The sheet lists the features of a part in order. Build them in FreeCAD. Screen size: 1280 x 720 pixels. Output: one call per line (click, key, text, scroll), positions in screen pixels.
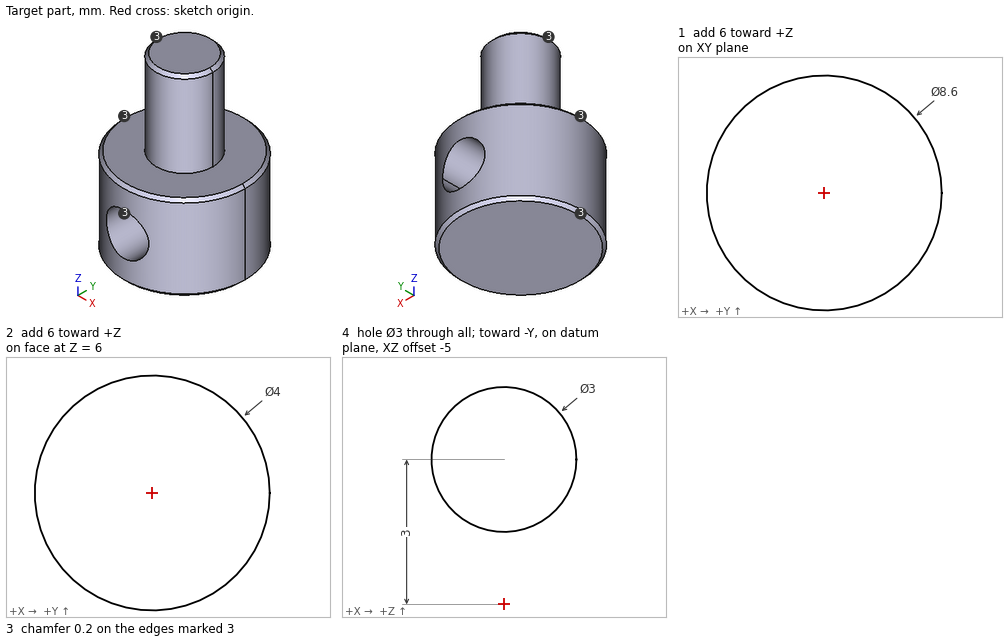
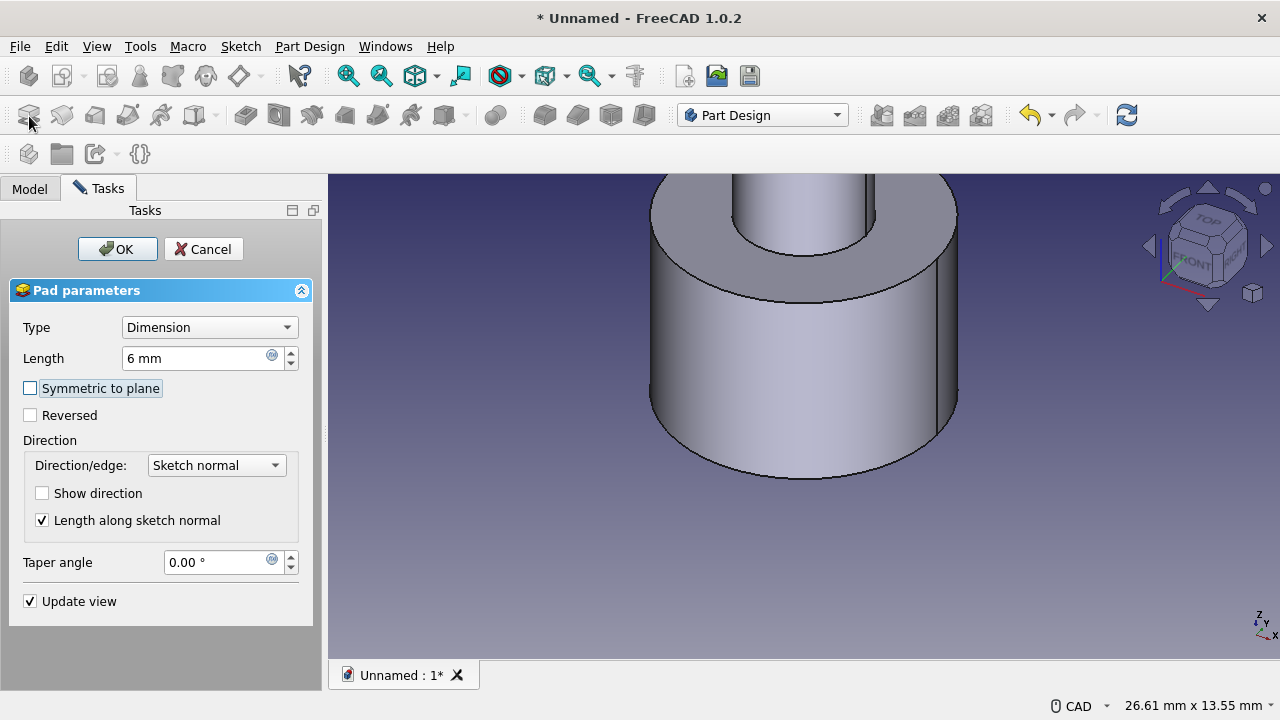
click(118, 249)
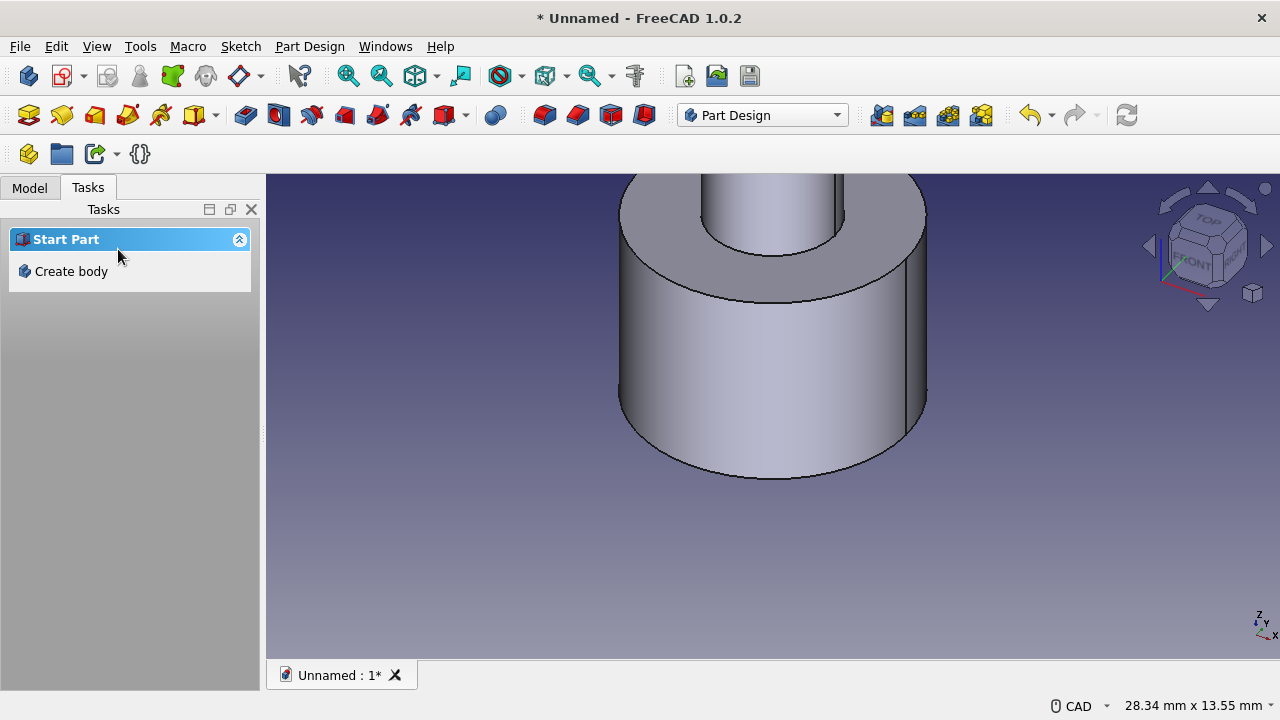
key(v)
key(f)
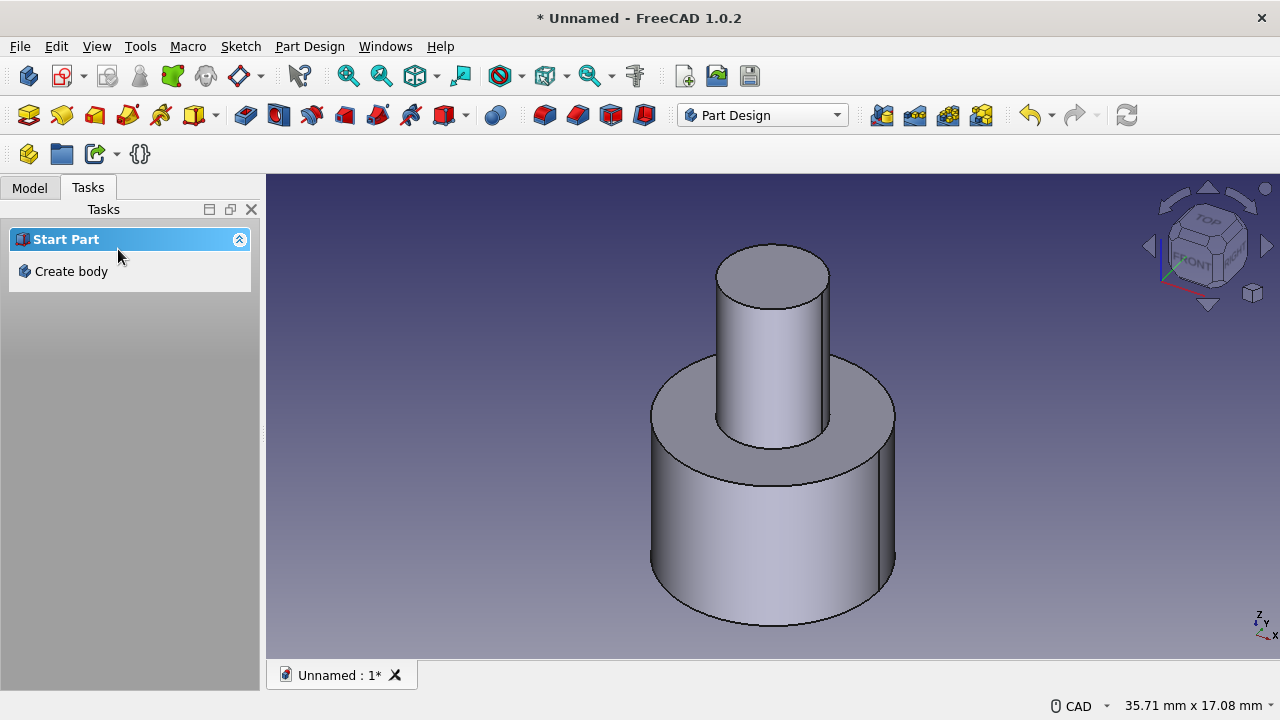
click(651, 423)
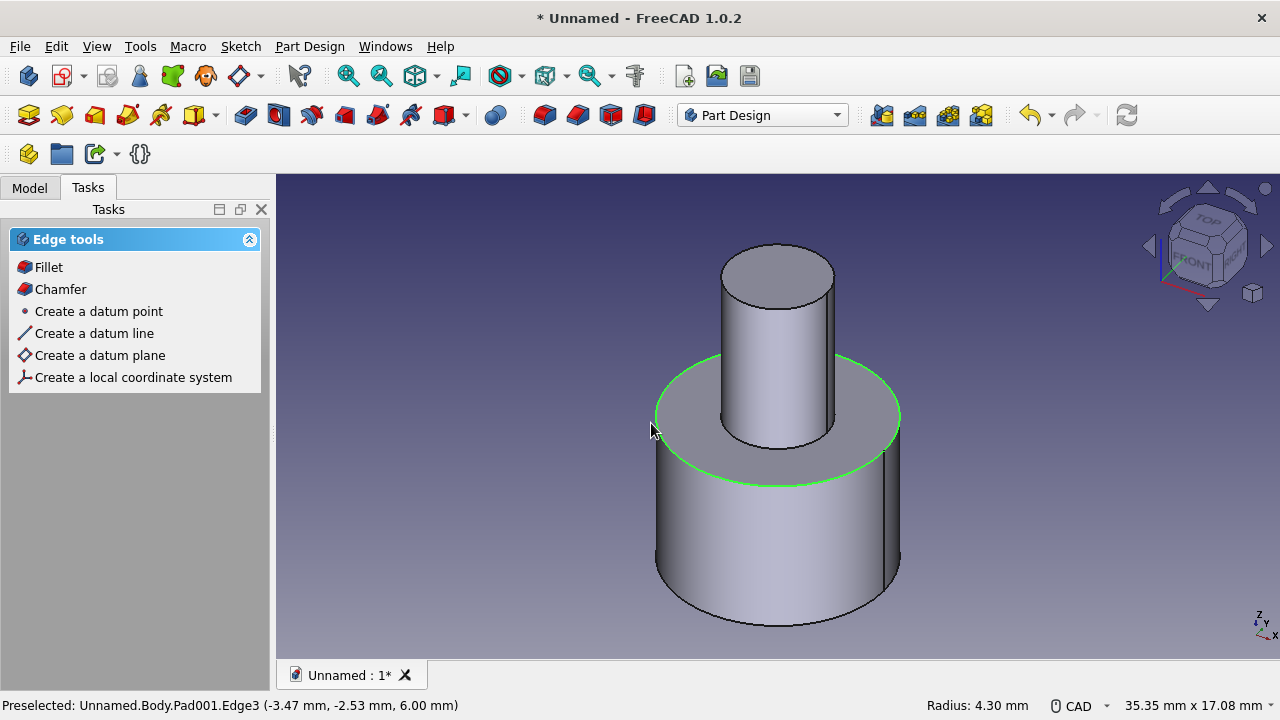
click(721, 279, ctrl)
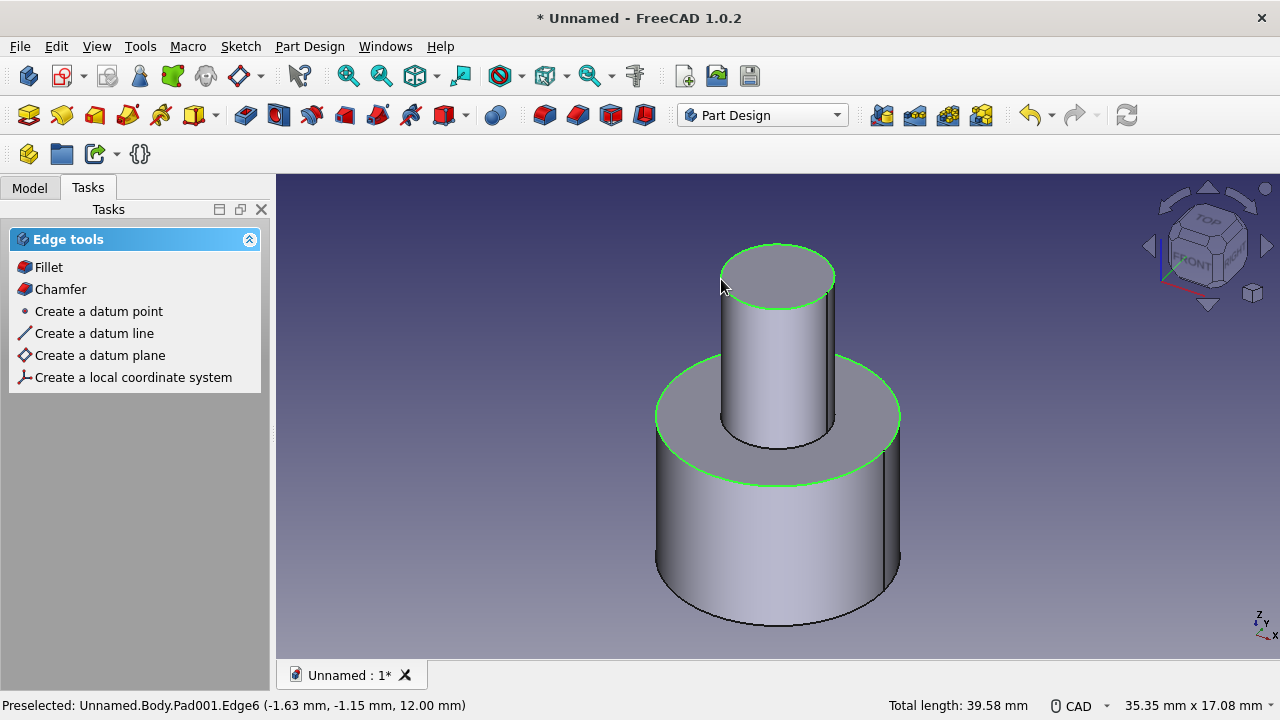
key(0)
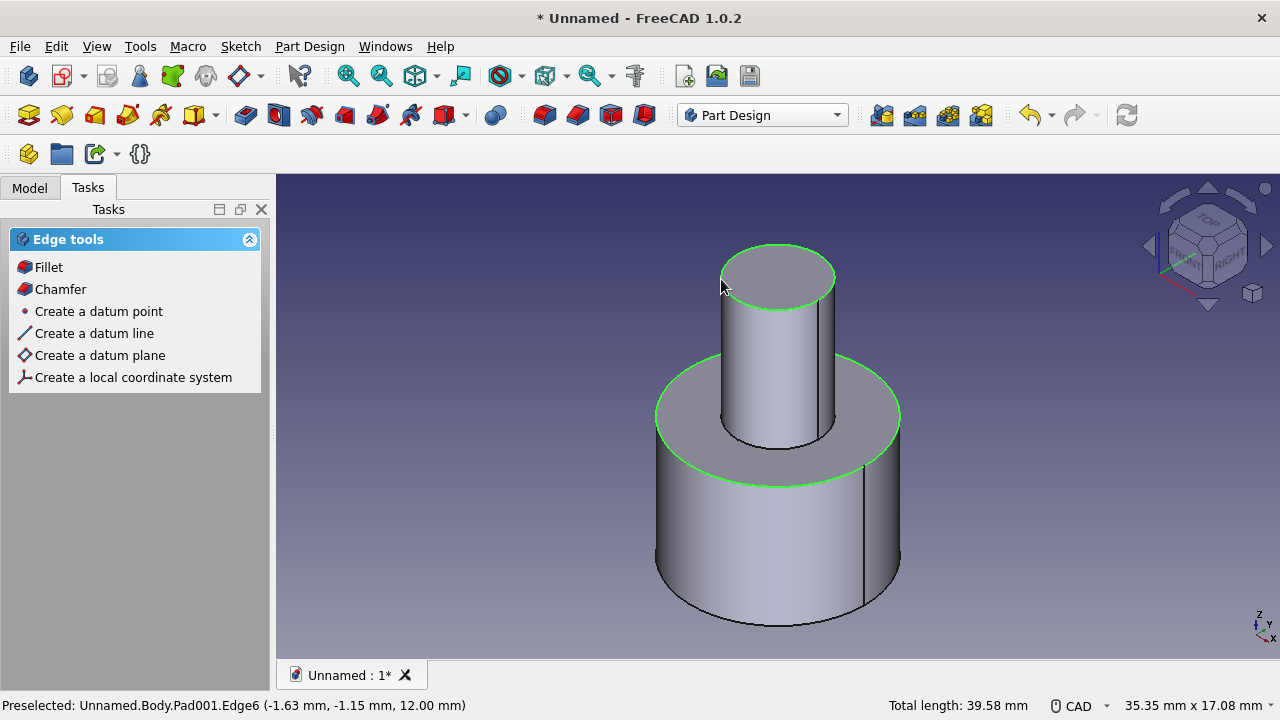
key(2)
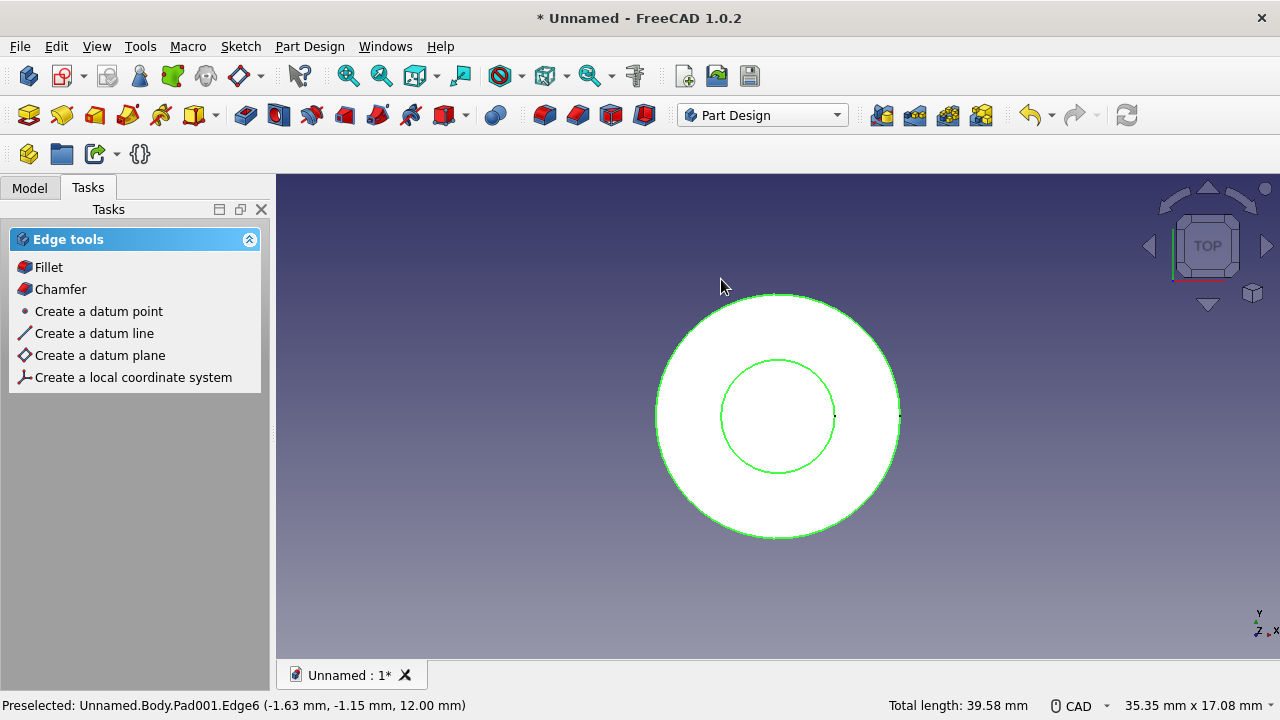
key(1)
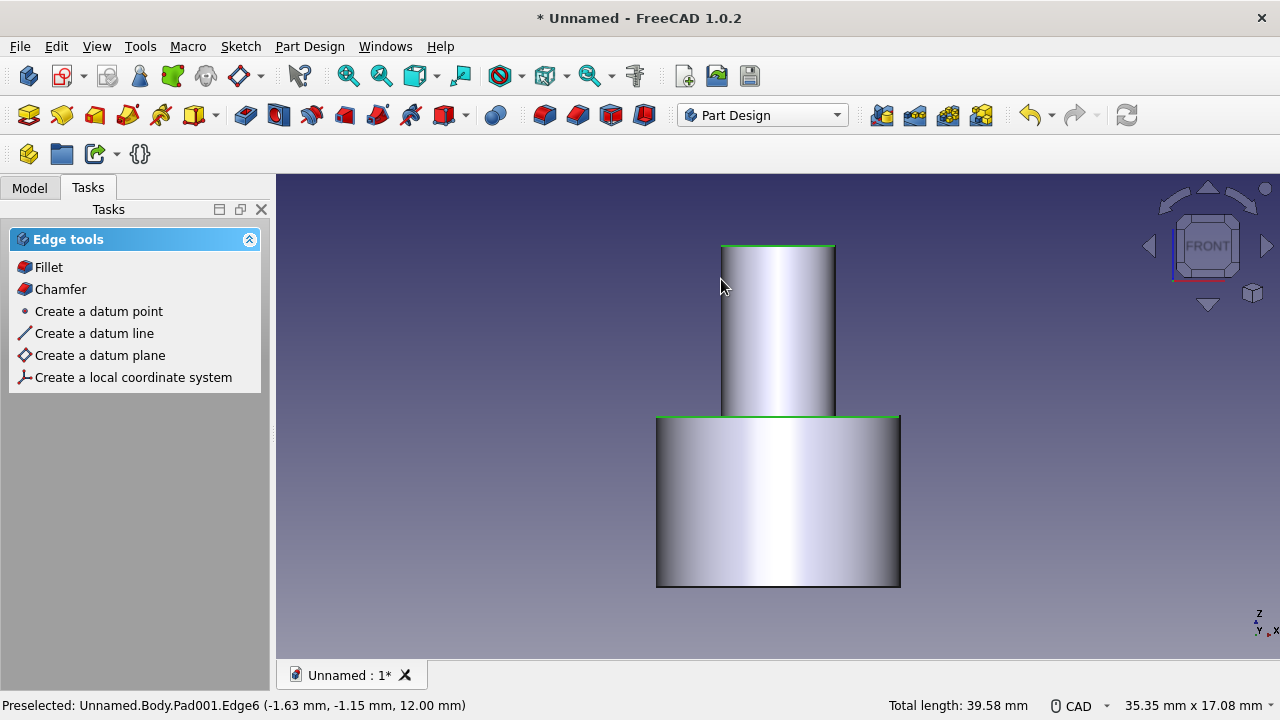
click(679, 586, ctrl)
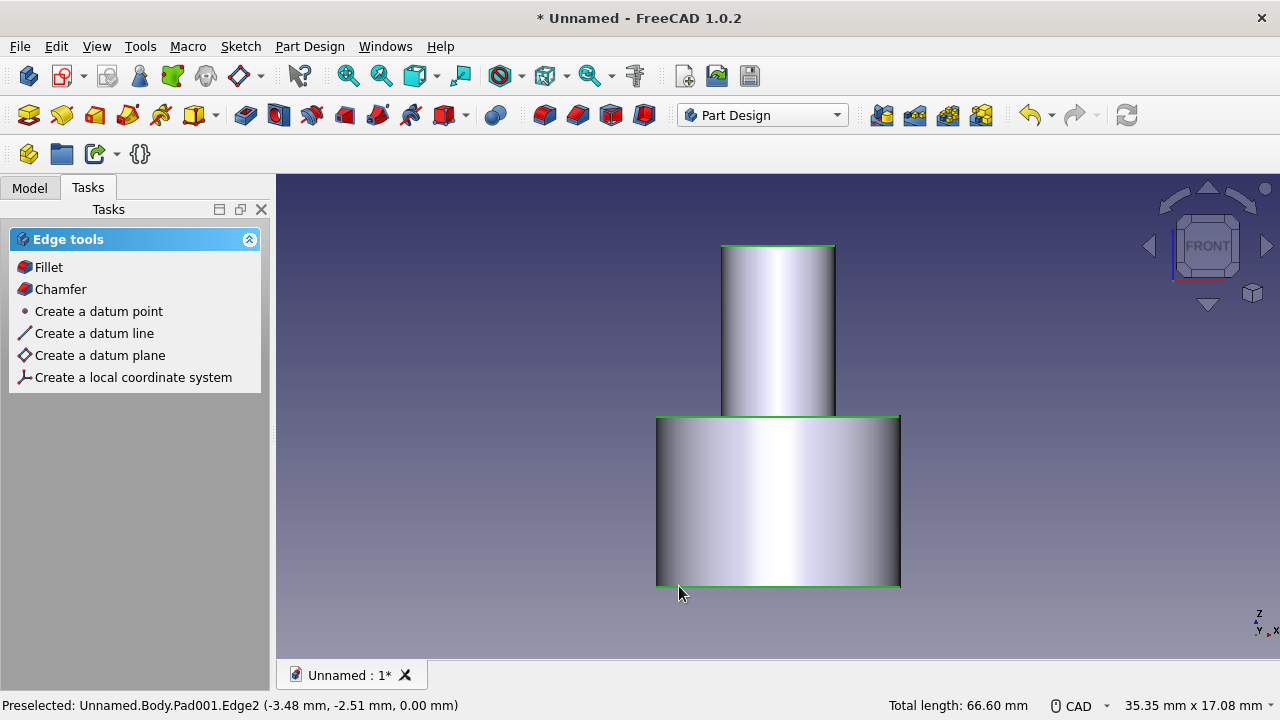
click(578, 116)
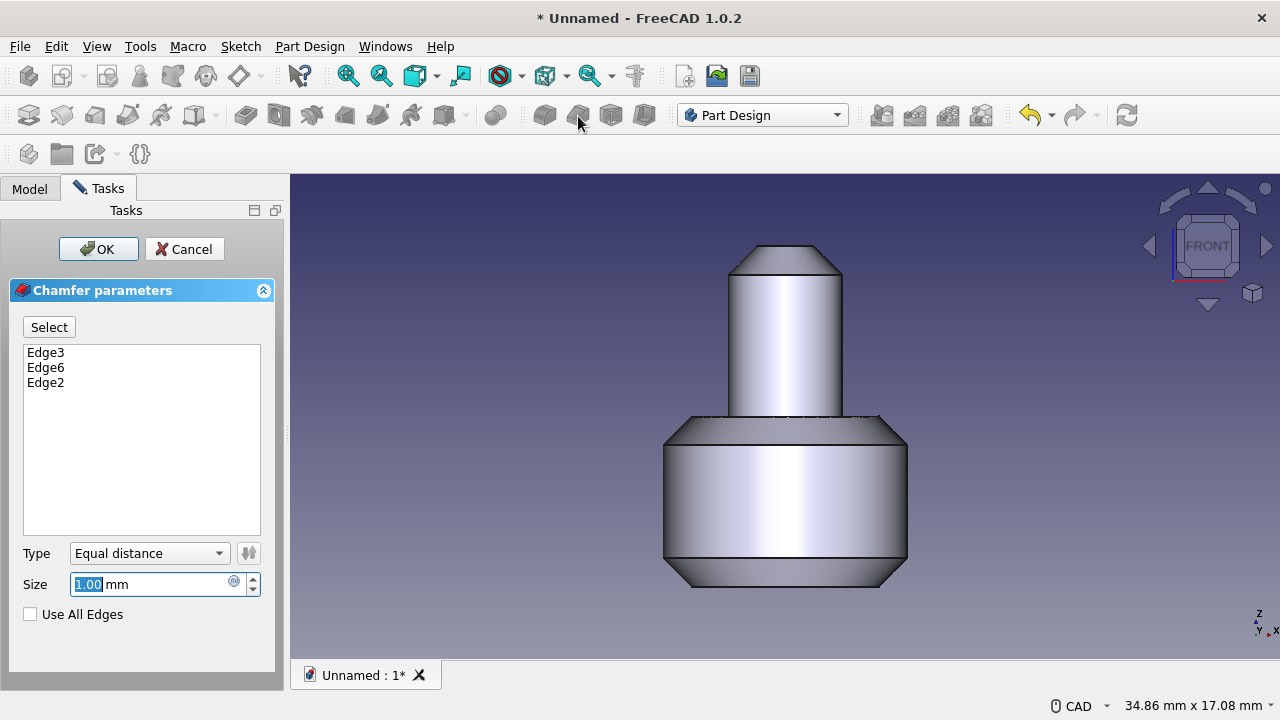
text(0.2)
key(Tab)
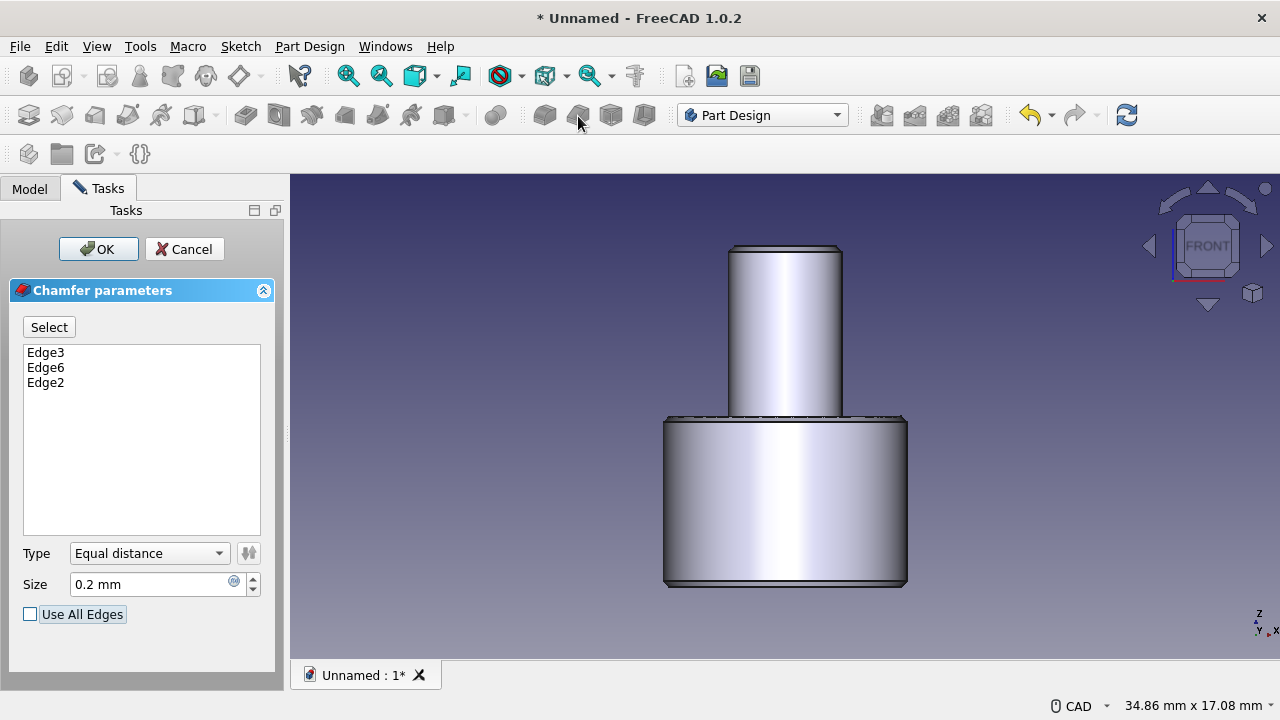
click(99, 249)